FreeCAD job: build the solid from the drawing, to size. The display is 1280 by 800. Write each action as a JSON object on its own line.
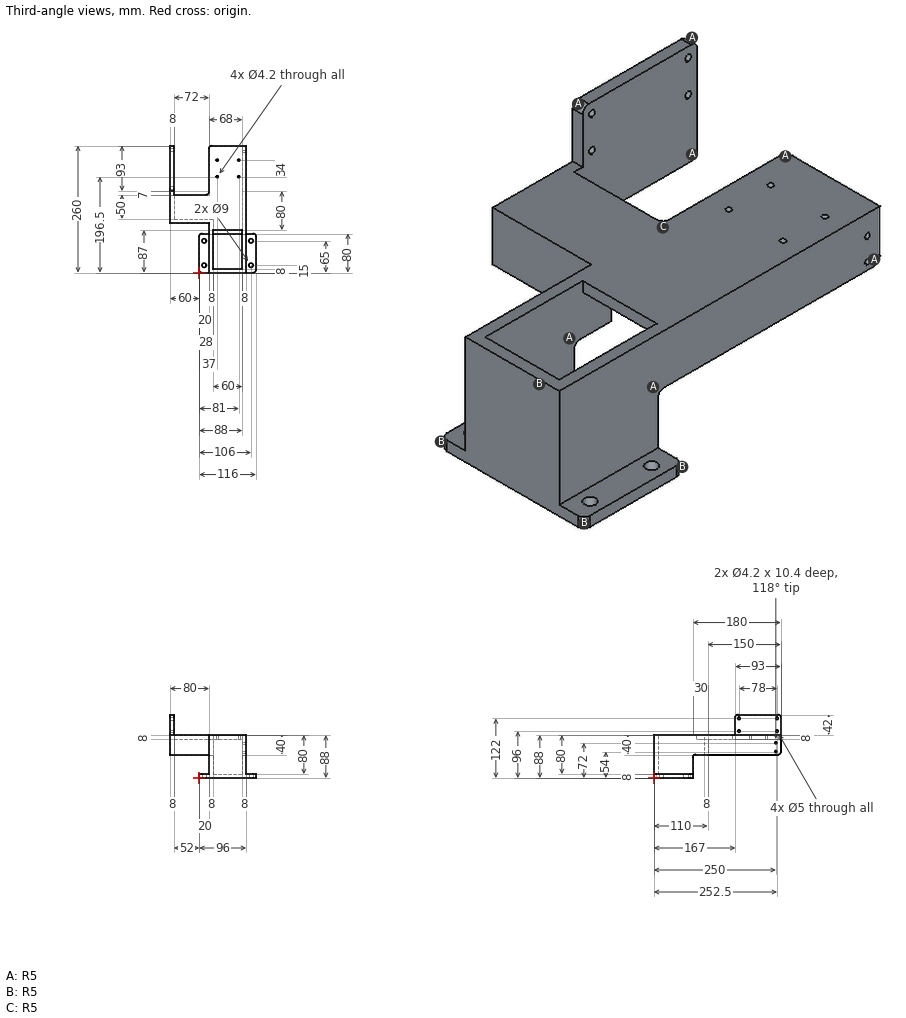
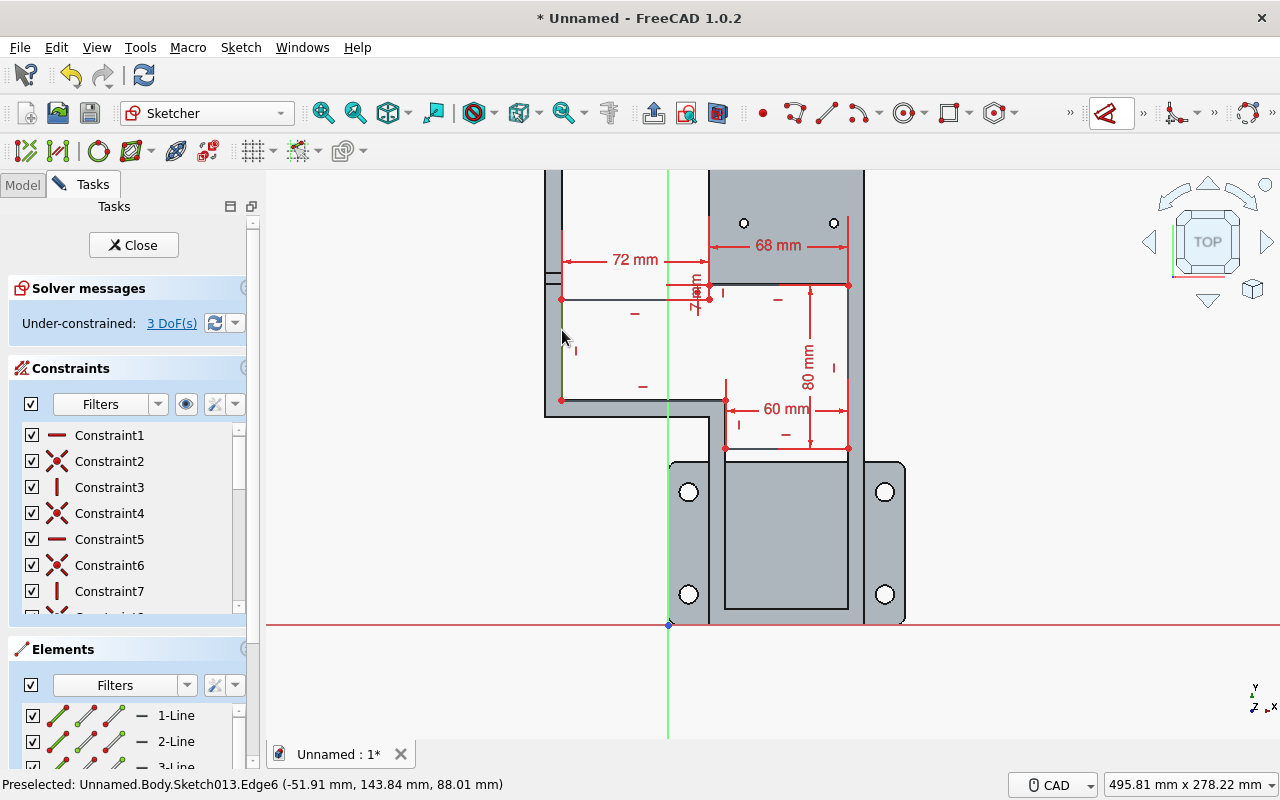
{"action": "left_click", "coordinate": [1128, 114]}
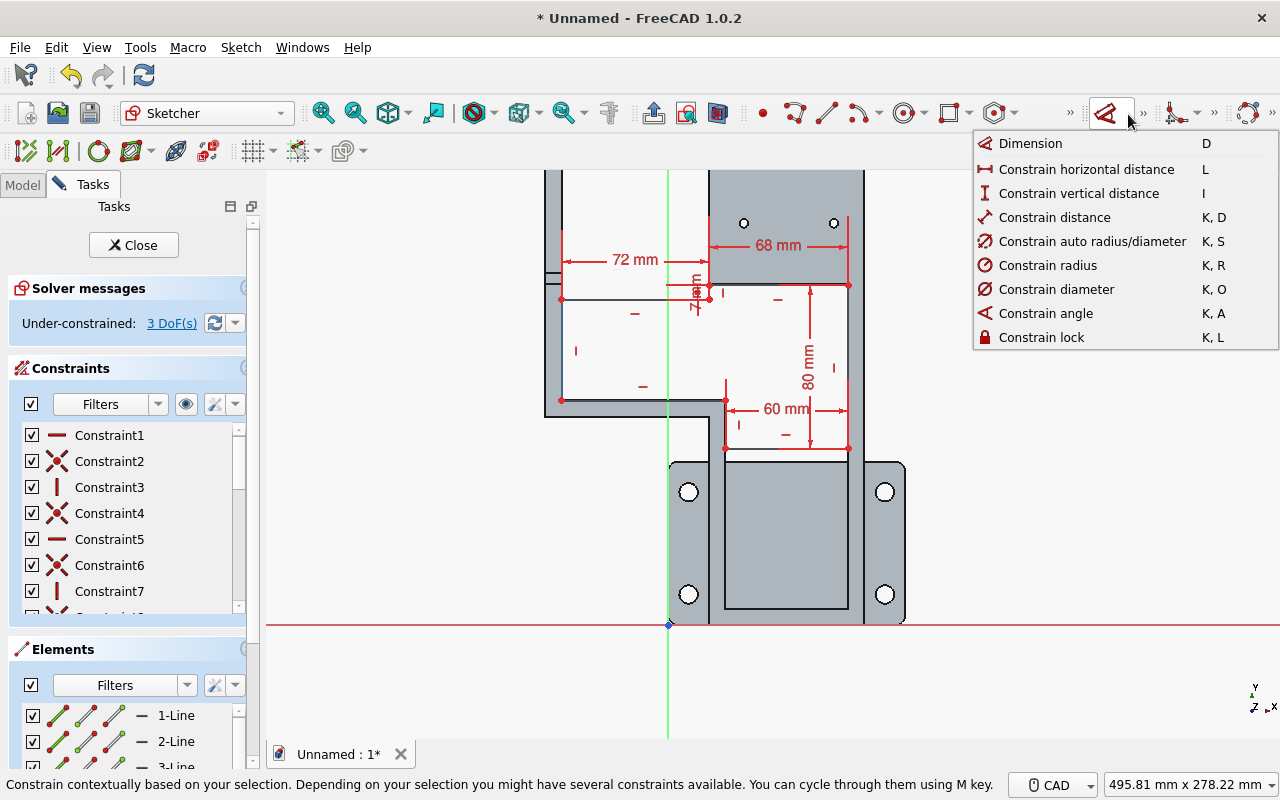
{"action": "left_click", "coordinate": [1126, 193]}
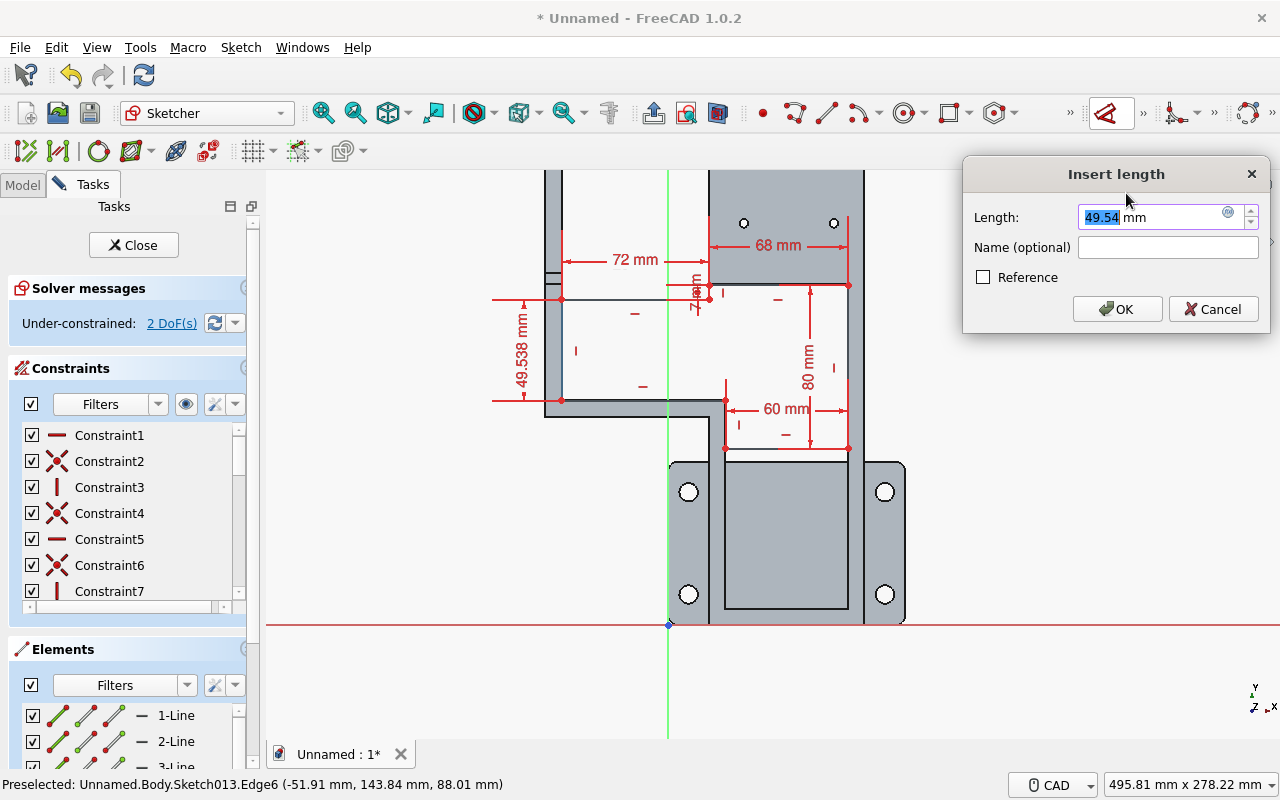
{"action": "type", "text": "50"}
{"action": "key", "text": "Return"}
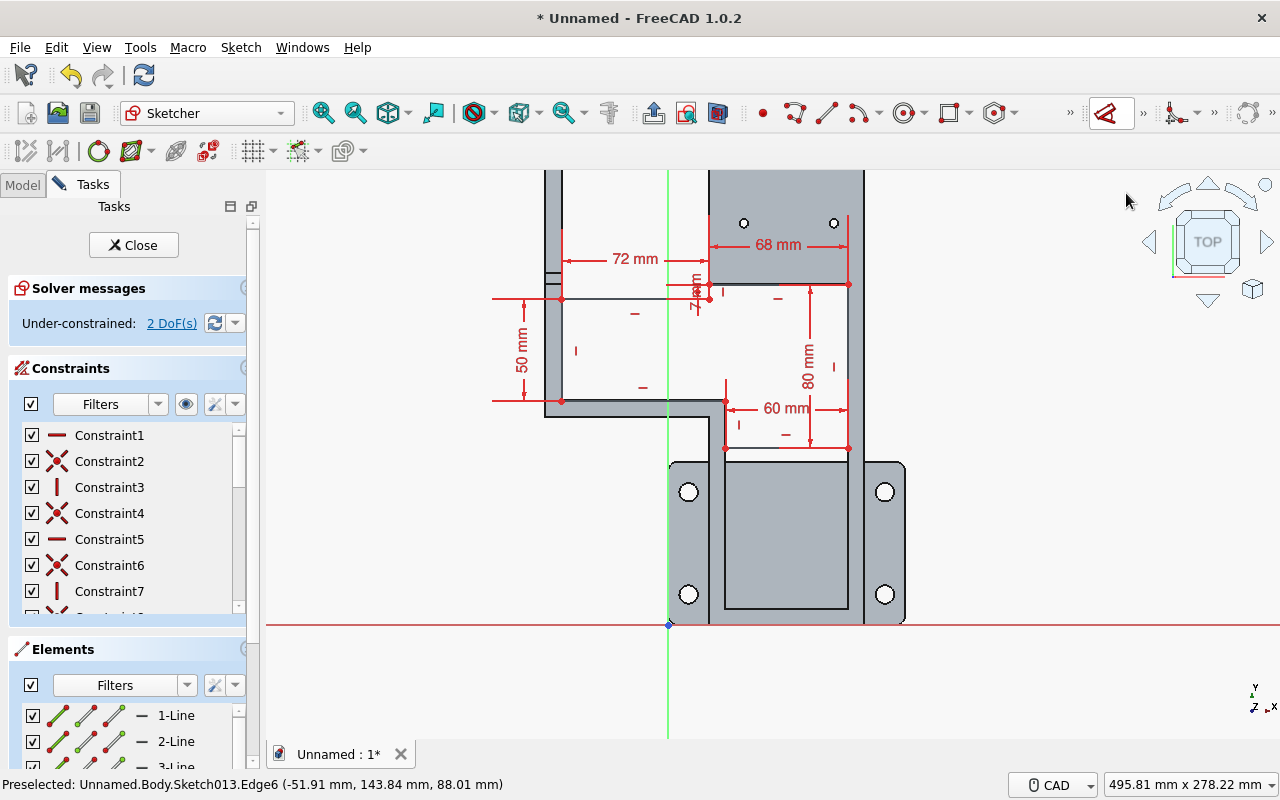
{"action": "left_click", "coordinate": [726, 448]}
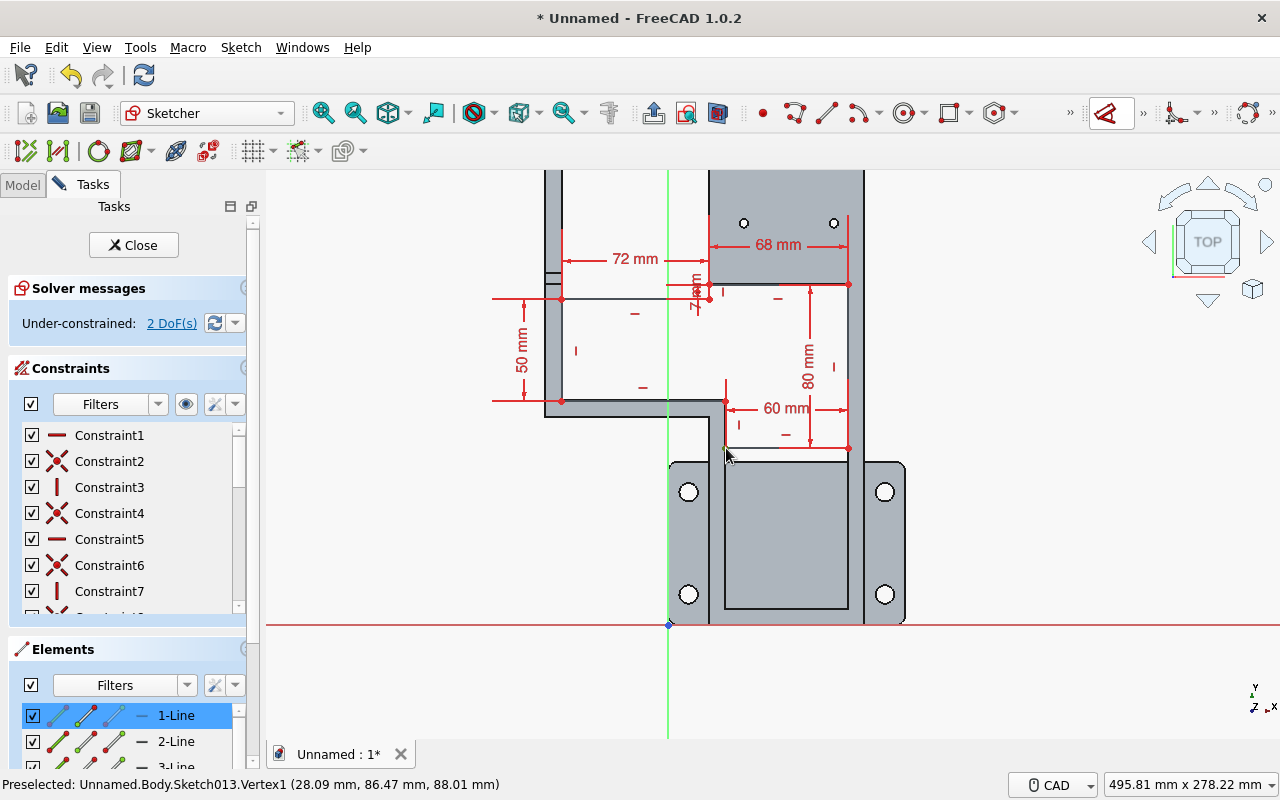
{"action": "left_click", "coordinate": [1128, 114]}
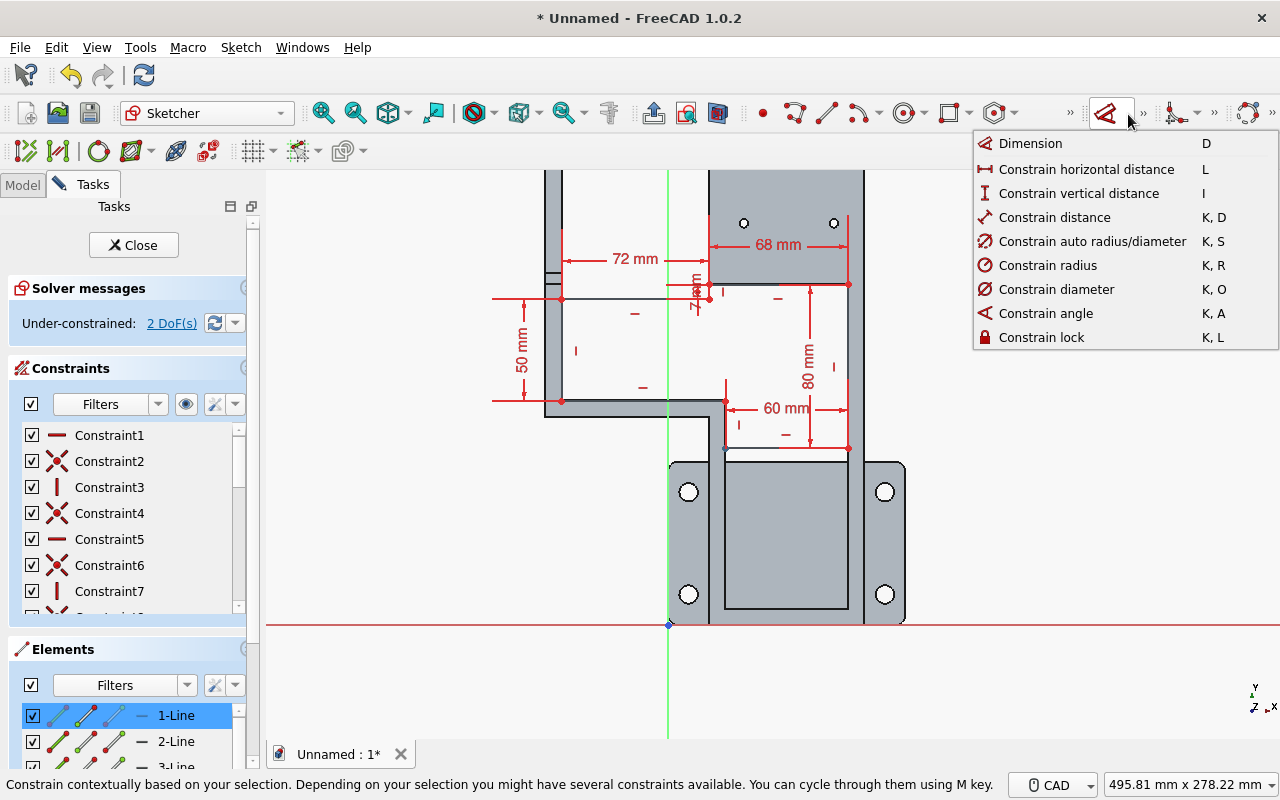
{"action": "left_click", "coordinate": [1126, 169]}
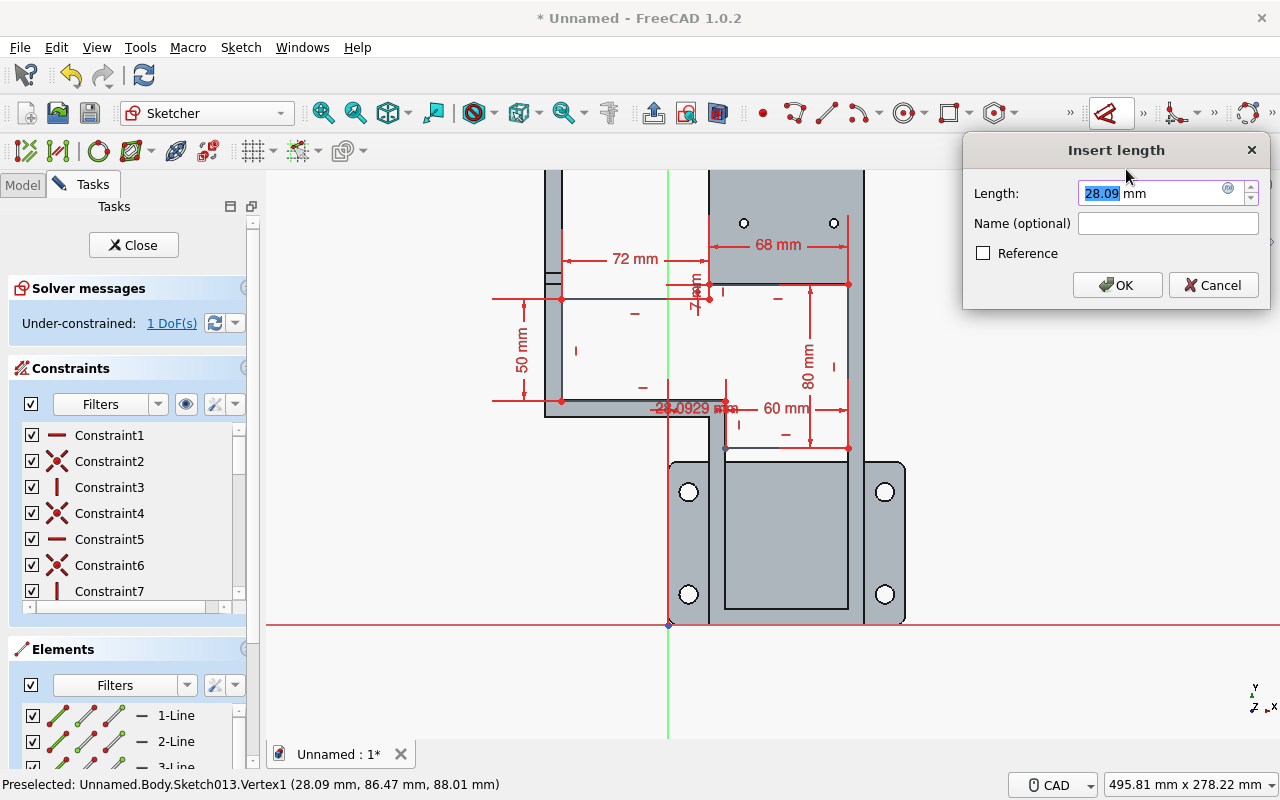
{"action": "type", "text": "28"}
{"action": "key", "text": "Return"}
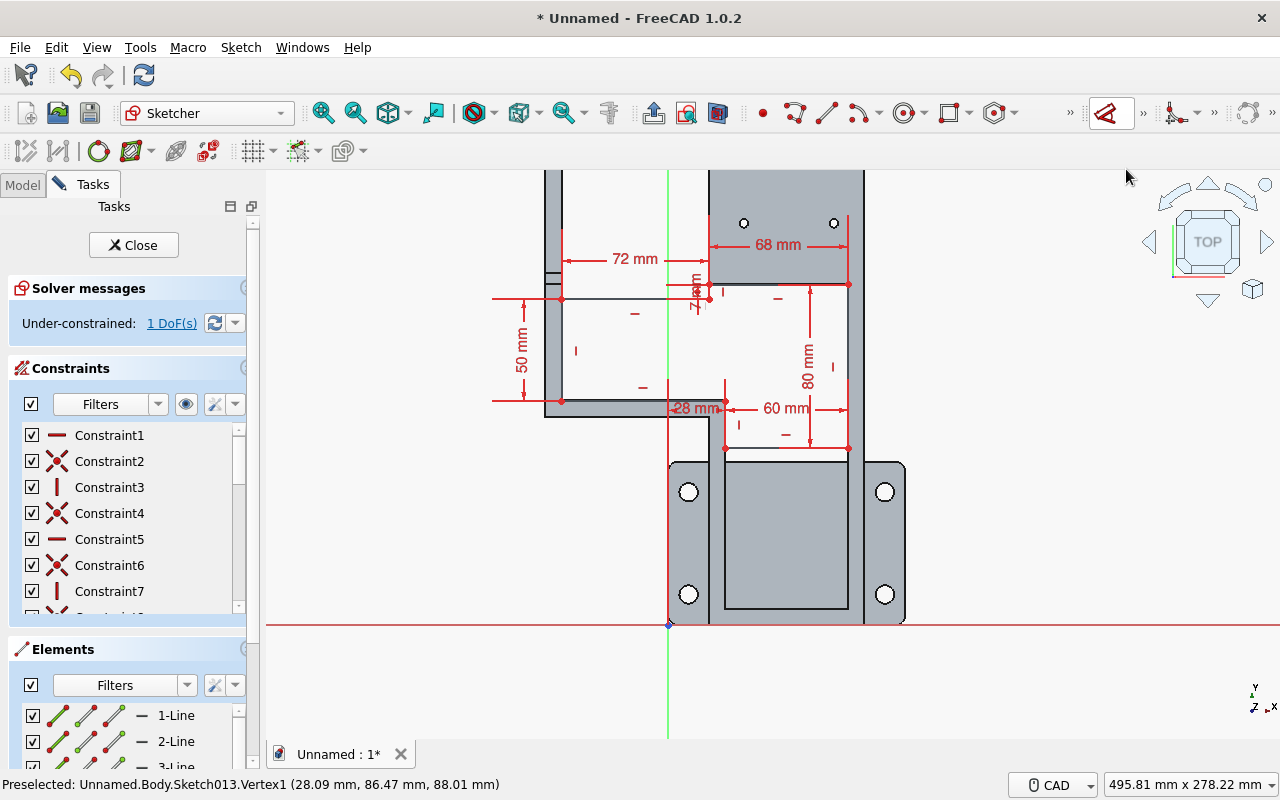
{"action": "left_click", "coordinate": [725, 448]}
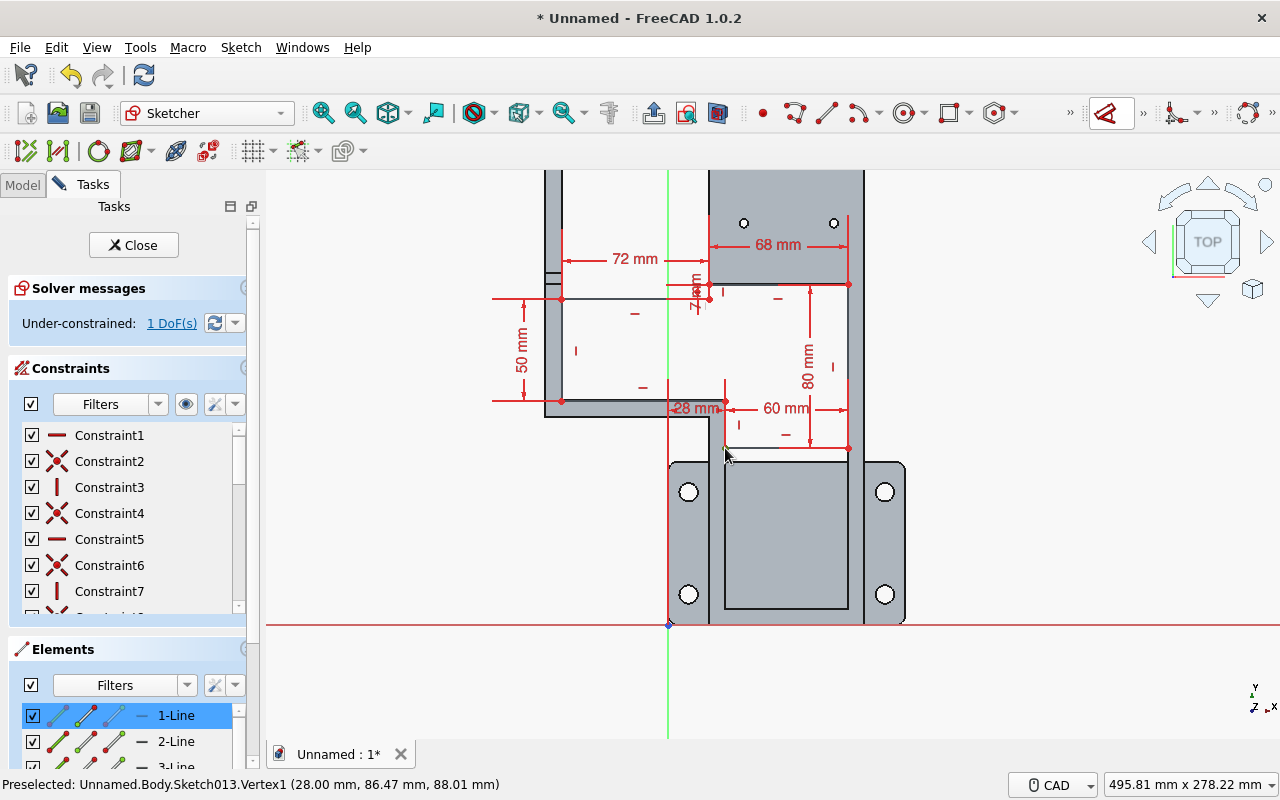
{"action": "left_click", "coordinate": [1128, 114]}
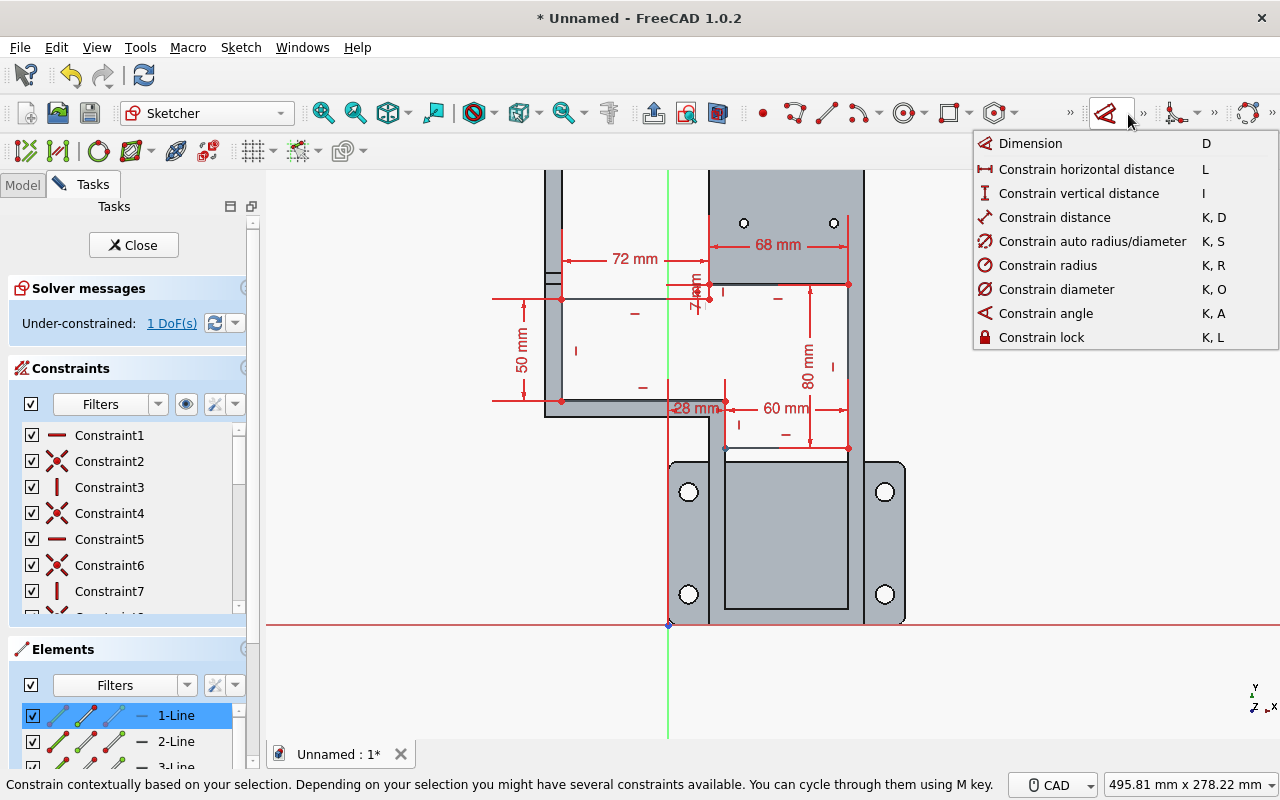
{"action": "left_click", "coordinate": [1126, 193]}